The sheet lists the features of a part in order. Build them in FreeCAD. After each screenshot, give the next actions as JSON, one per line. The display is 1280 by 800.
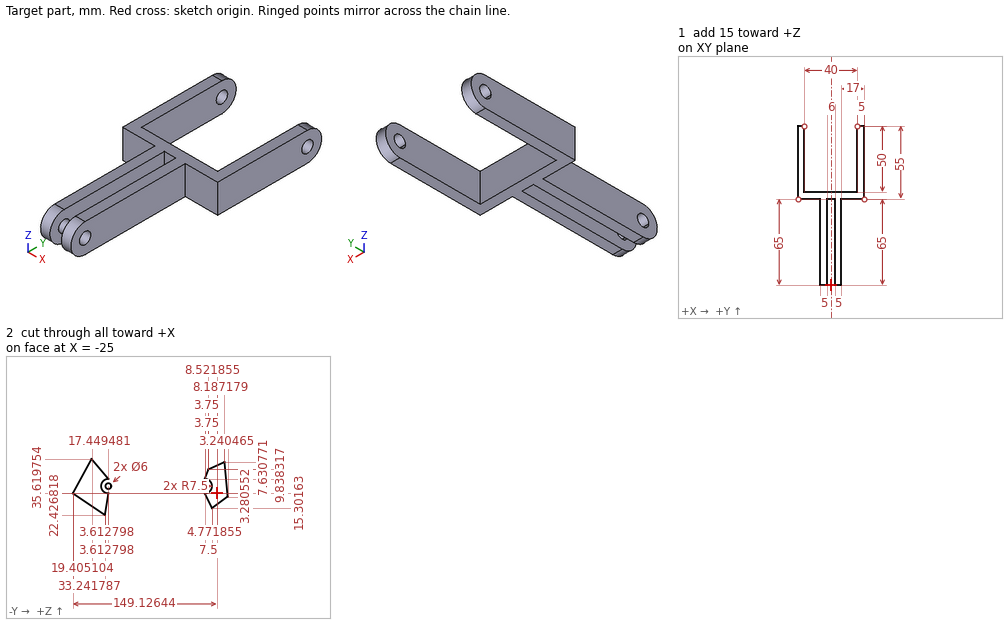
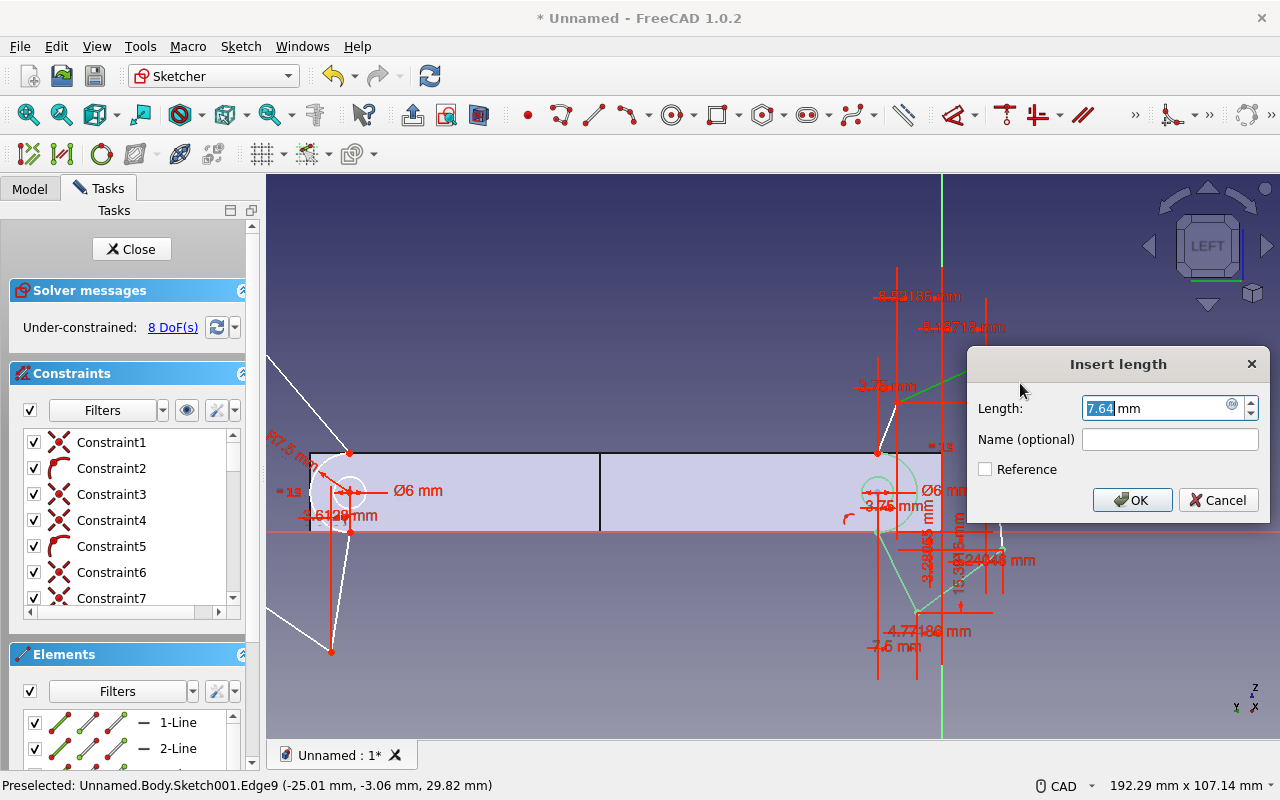
{"action": "type", "text": "7.630771"}
{"action": "key", "text": "Return"}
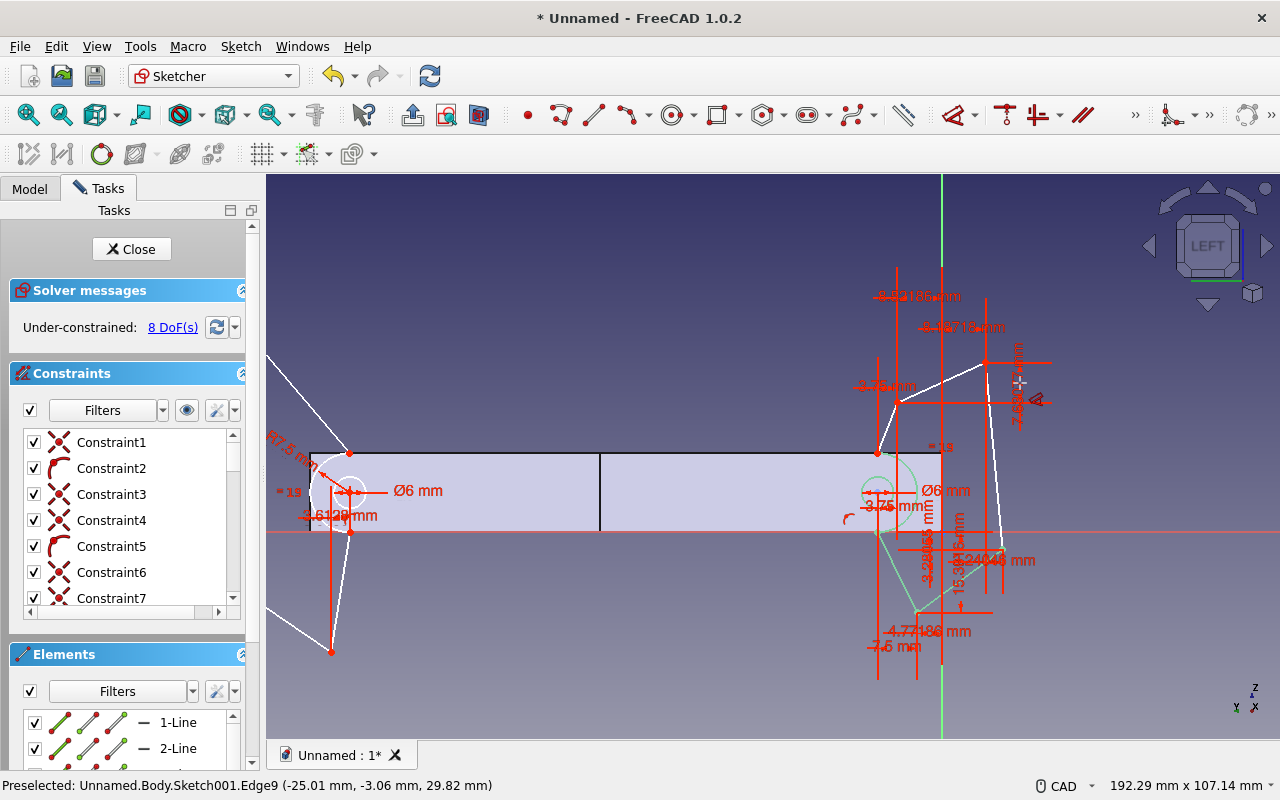
{"action": "left_click", "coordinate": [892, 418]}
{"action": "left_click", "coordinate": [844, 428]}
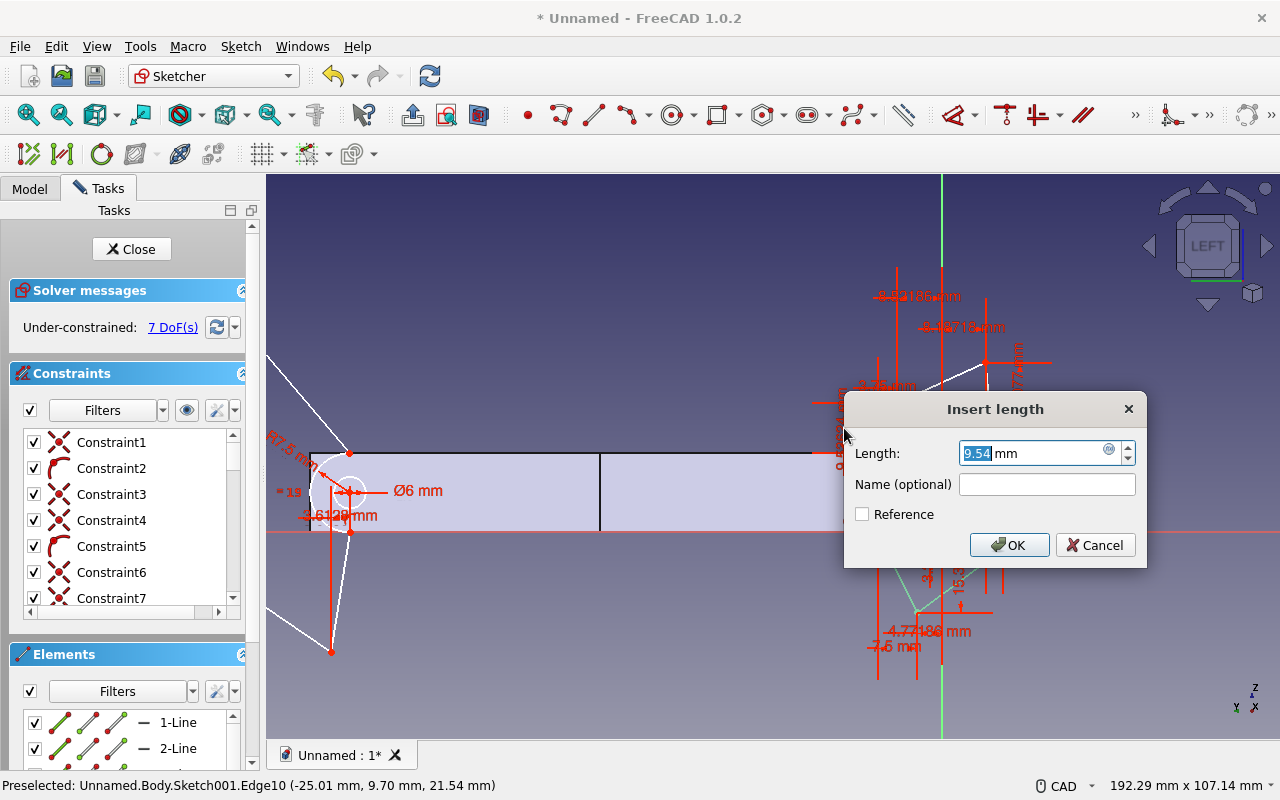
{"action": "type", "text": "9.838317"}
{"action": "key", "text": "Return"}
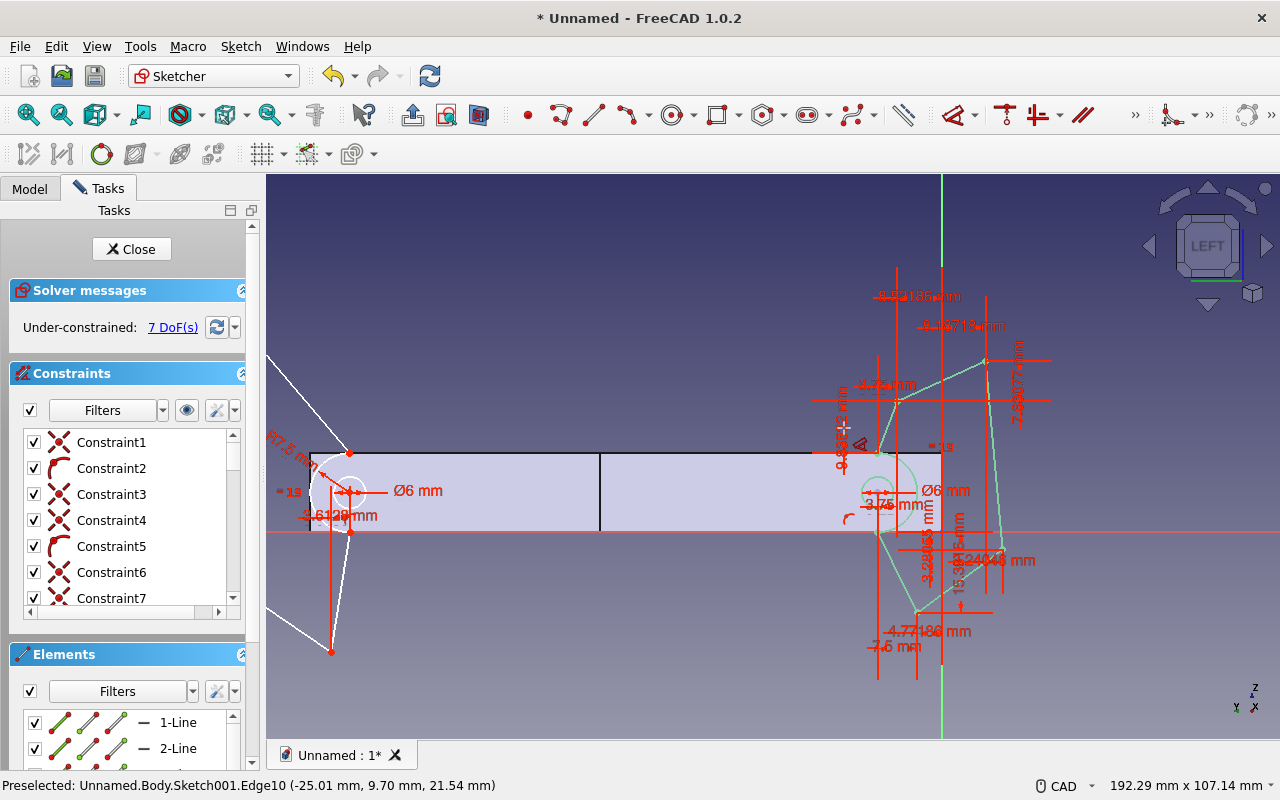
{"action": "scroll", "coordinate": [331, 652], "scroll_direction": "up", "scroll_amount": 4}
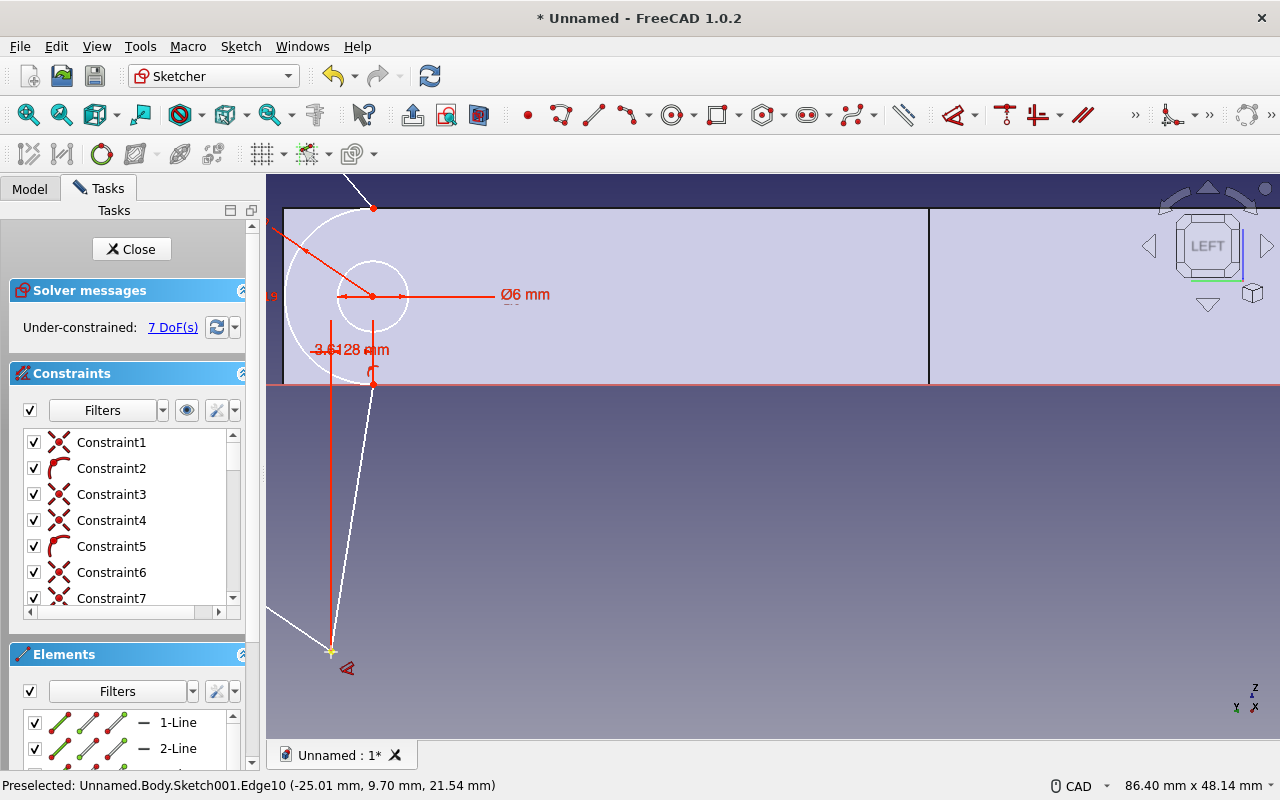
{"action": "left_click", "coordinate": [331, 651]}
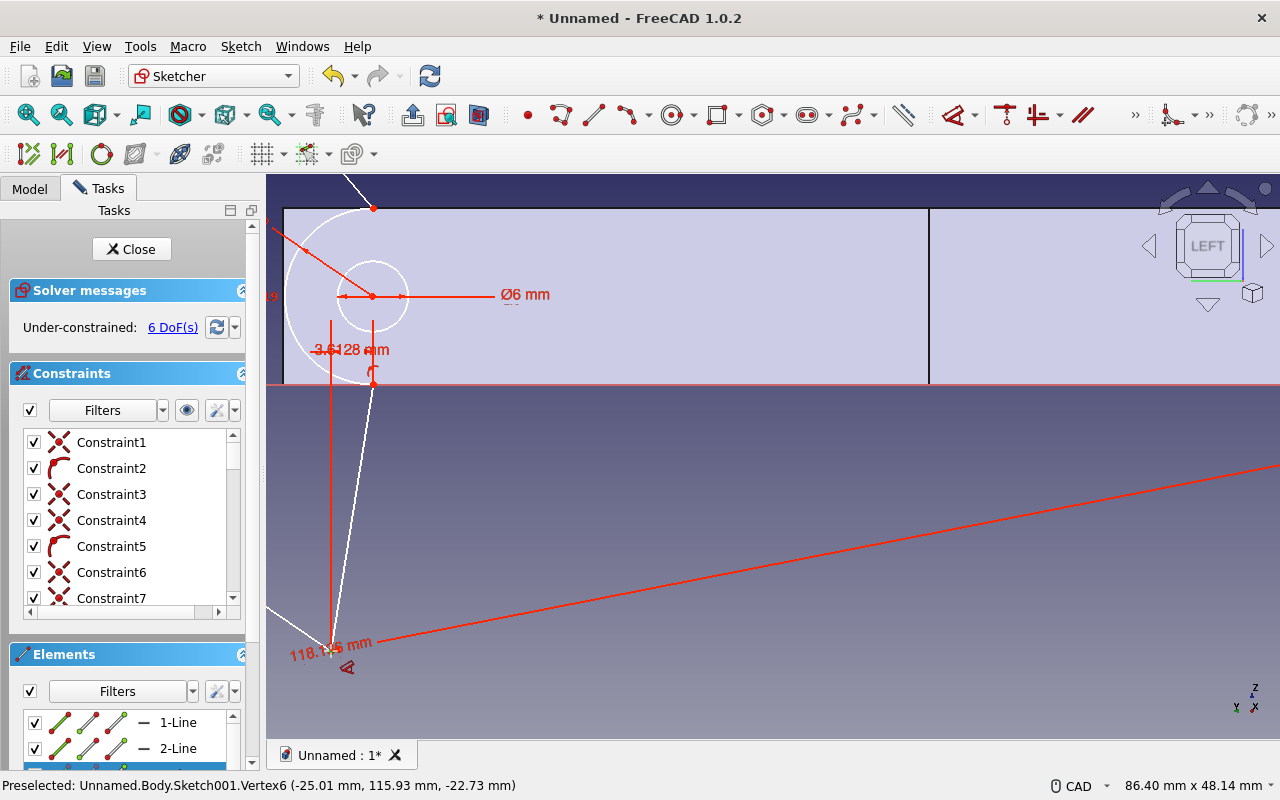
{"action": "left_click", "coordinate": [373, 297]}
{"action": "left_click", "coordinate": [352, 685]}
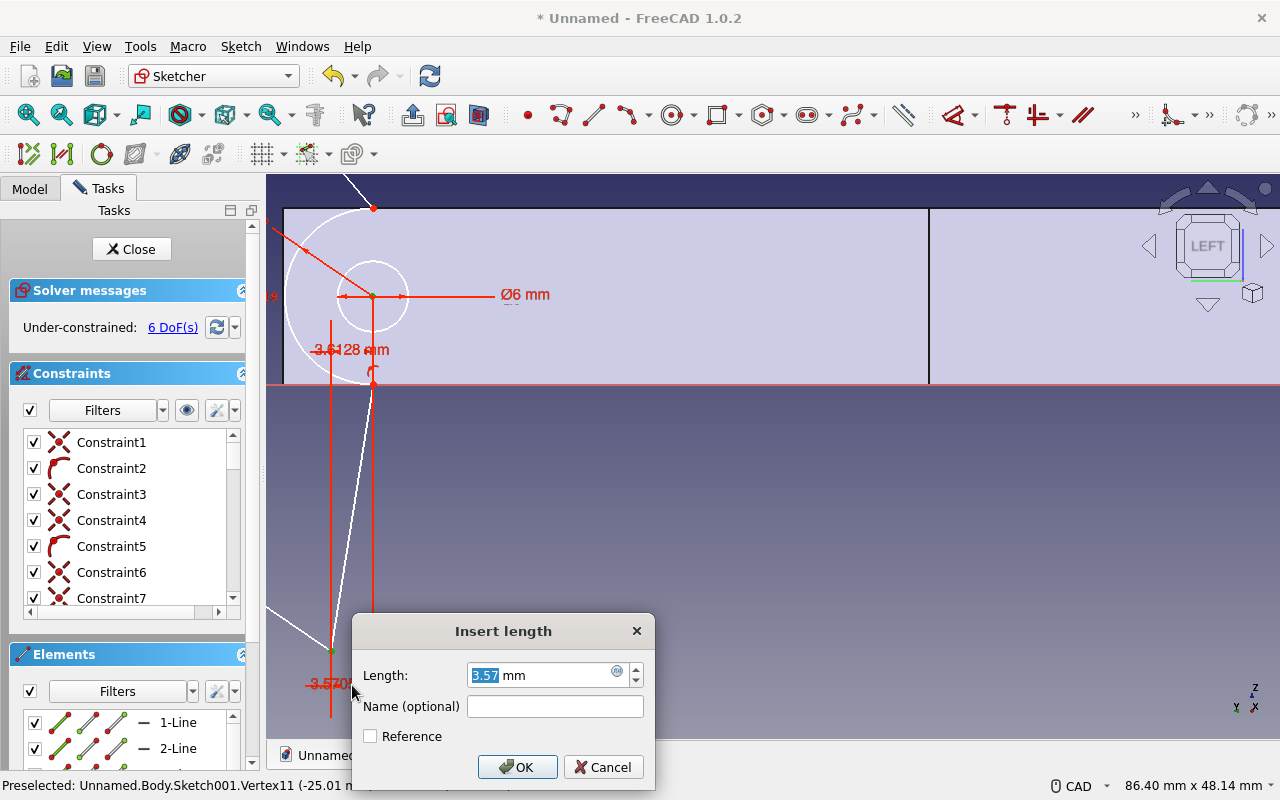
{"action": "type", "text": "3.612798"}
{"action": "key", "text": "Return"}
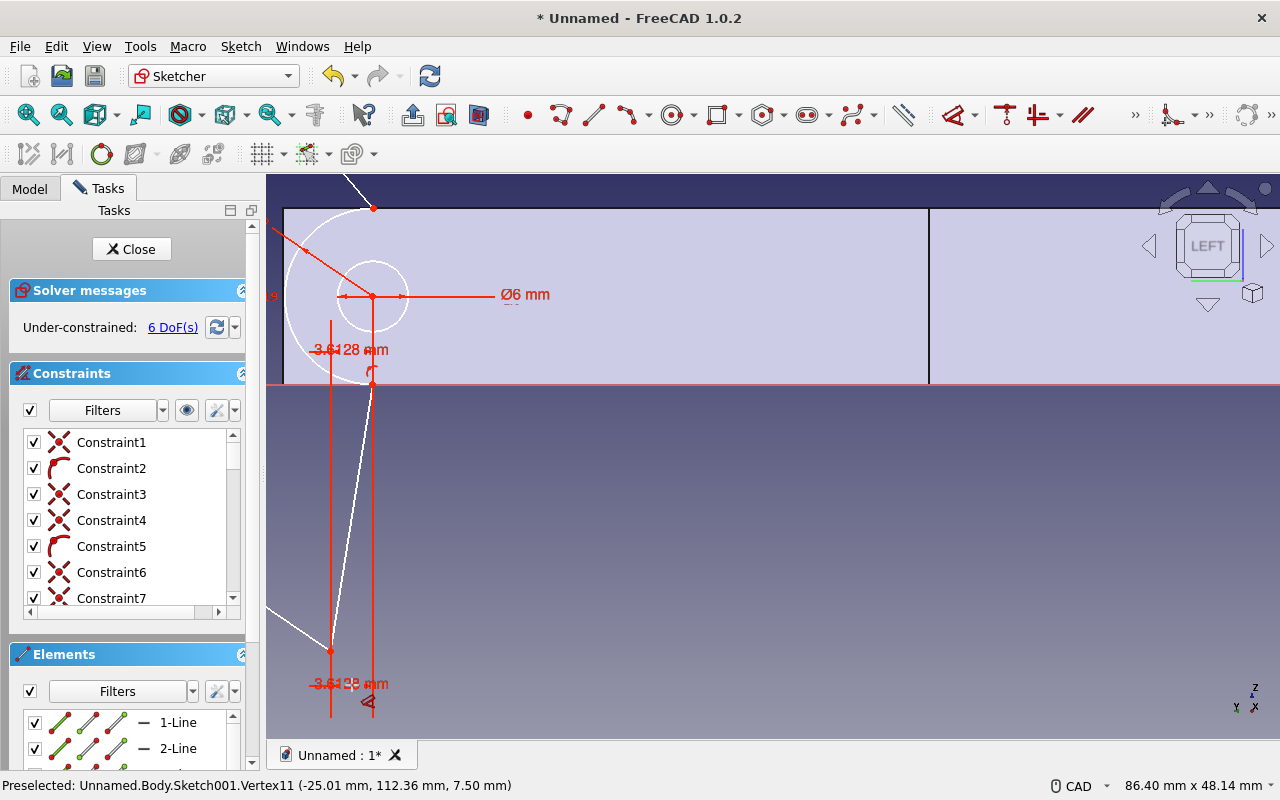
{"action": "scroll", "coordinate": [627, 521], "scroll_direction": "down", "scroll_amount": 6}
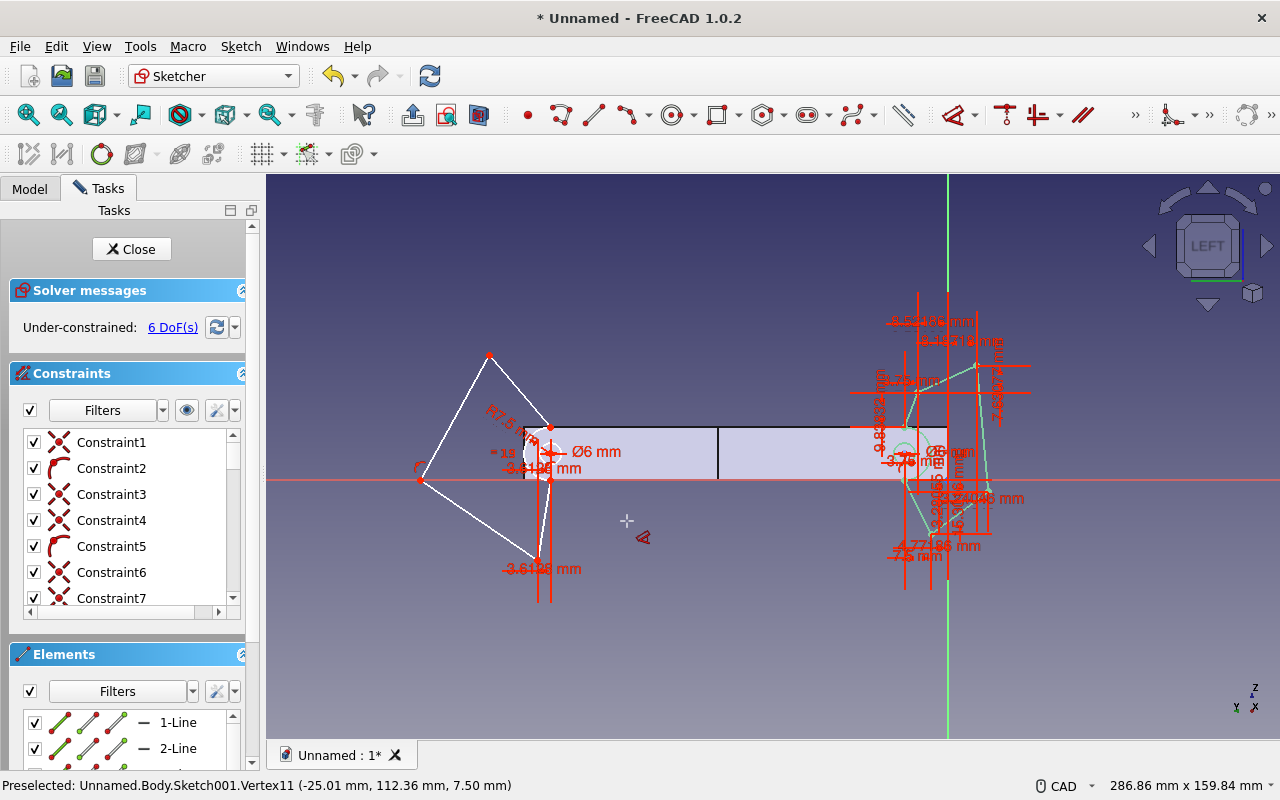
{"action": "left_click", "coordinate": [489, 355]}
{"action": "left_click", "coordinate": [455, 389]}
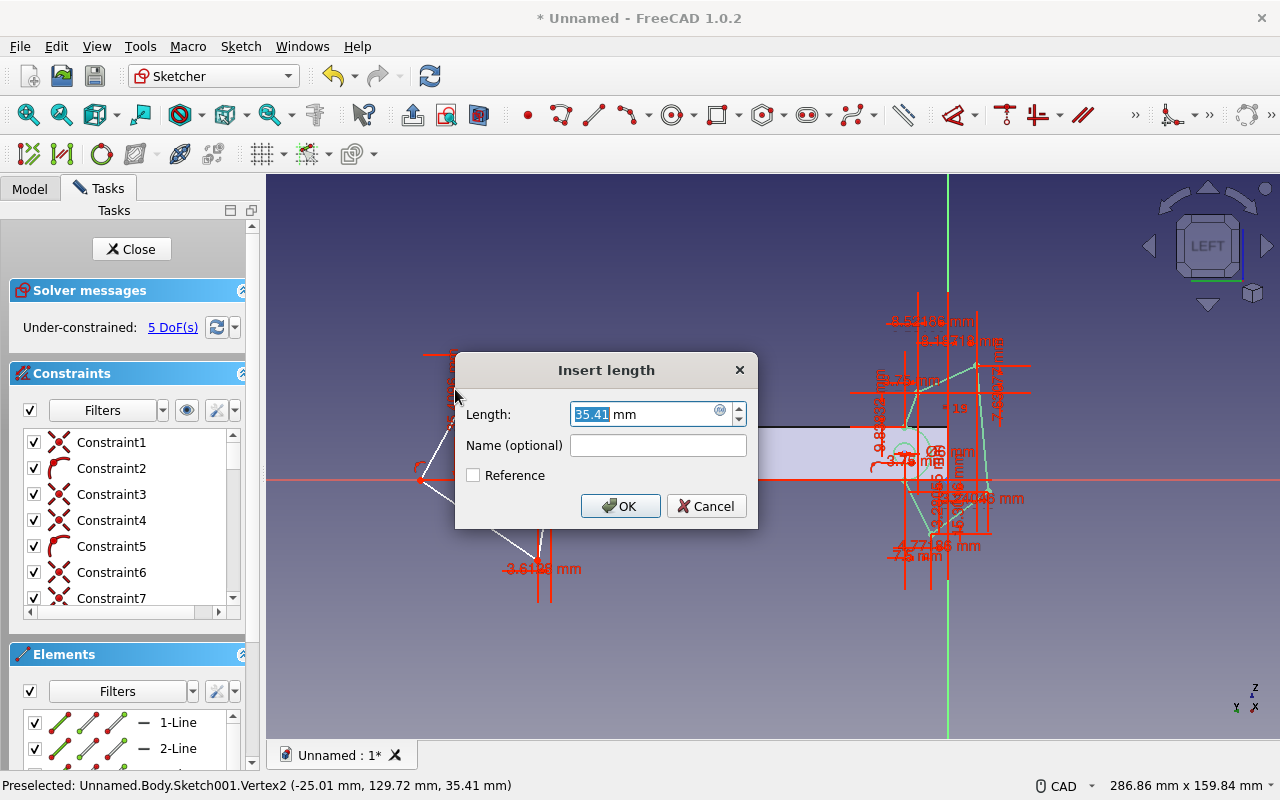
{"action": "type", "text": "35.619754"}
{"action": "key", "text": "Return"}